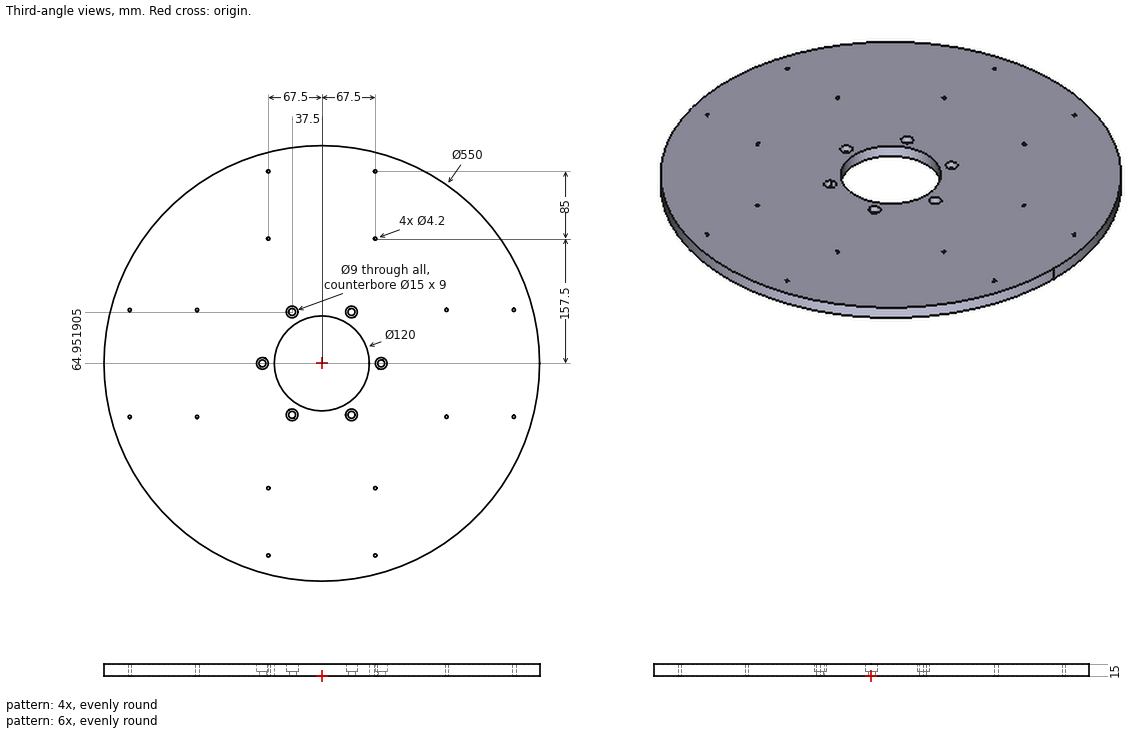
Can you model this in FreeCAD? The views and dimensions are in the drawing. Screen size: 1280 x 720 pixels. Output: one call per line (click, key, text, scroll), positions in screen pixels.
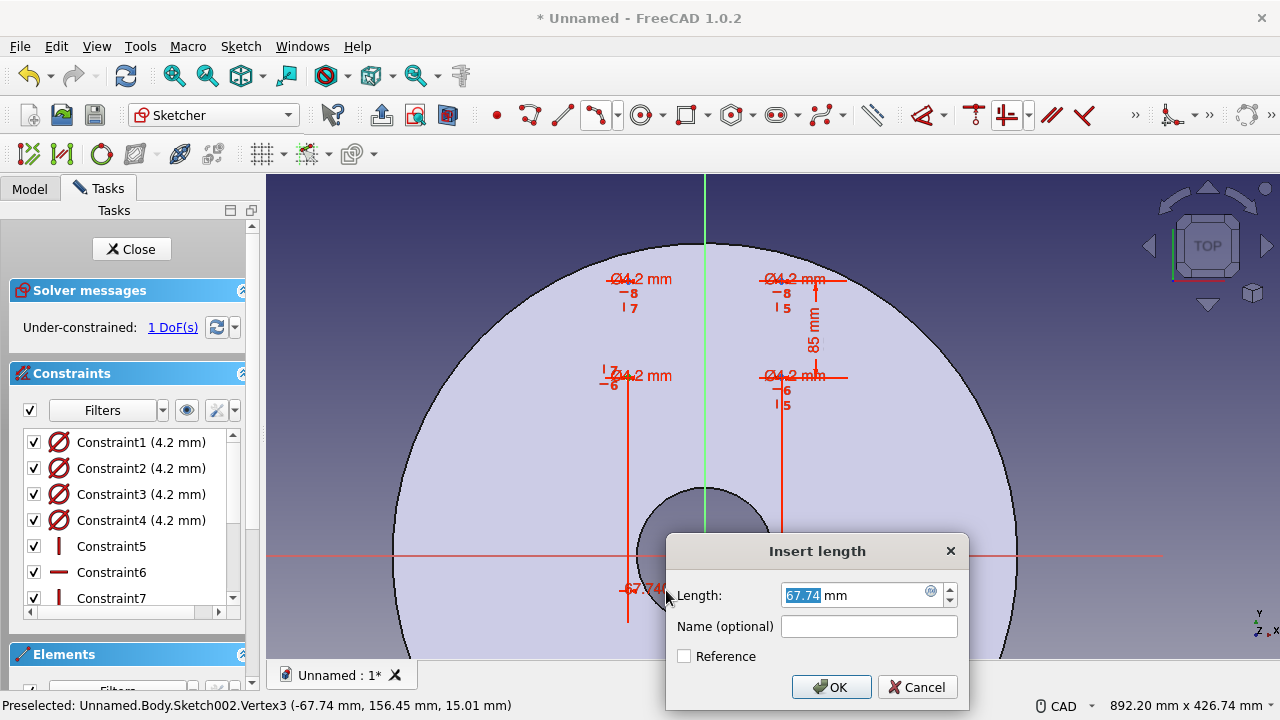
text(67.5)
key(Return)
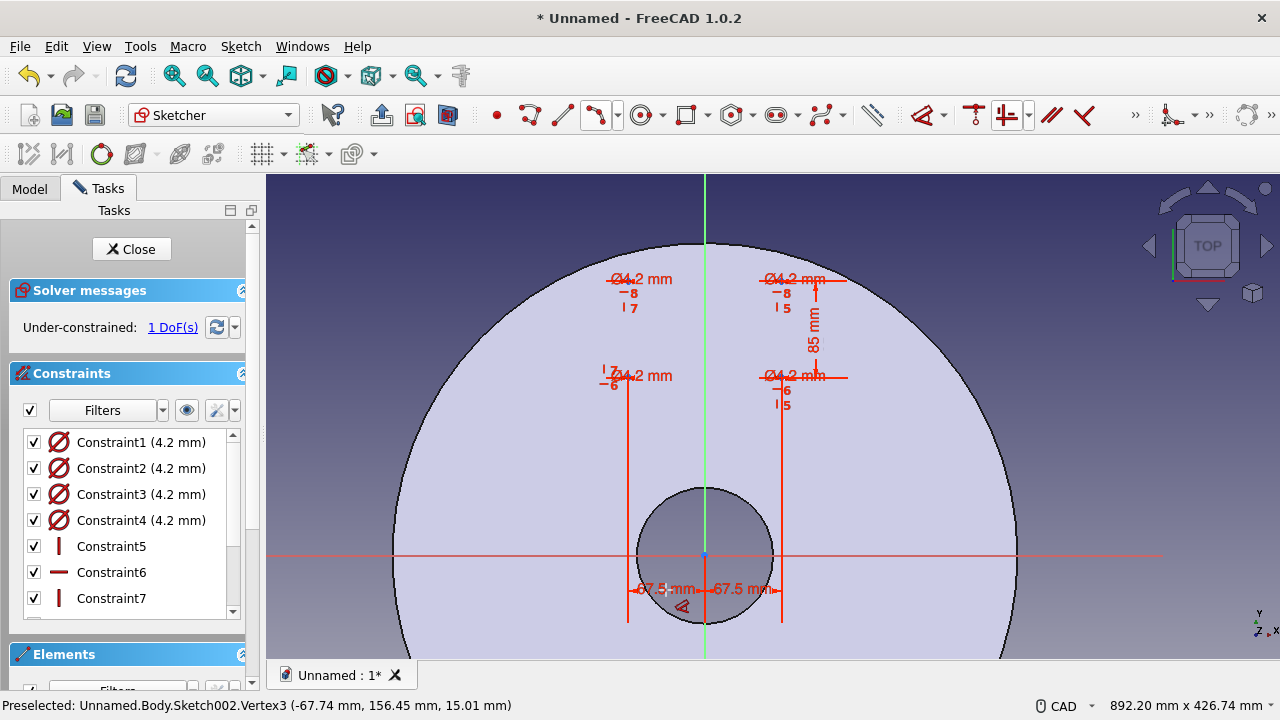
click(782, 378)
click(816, 467)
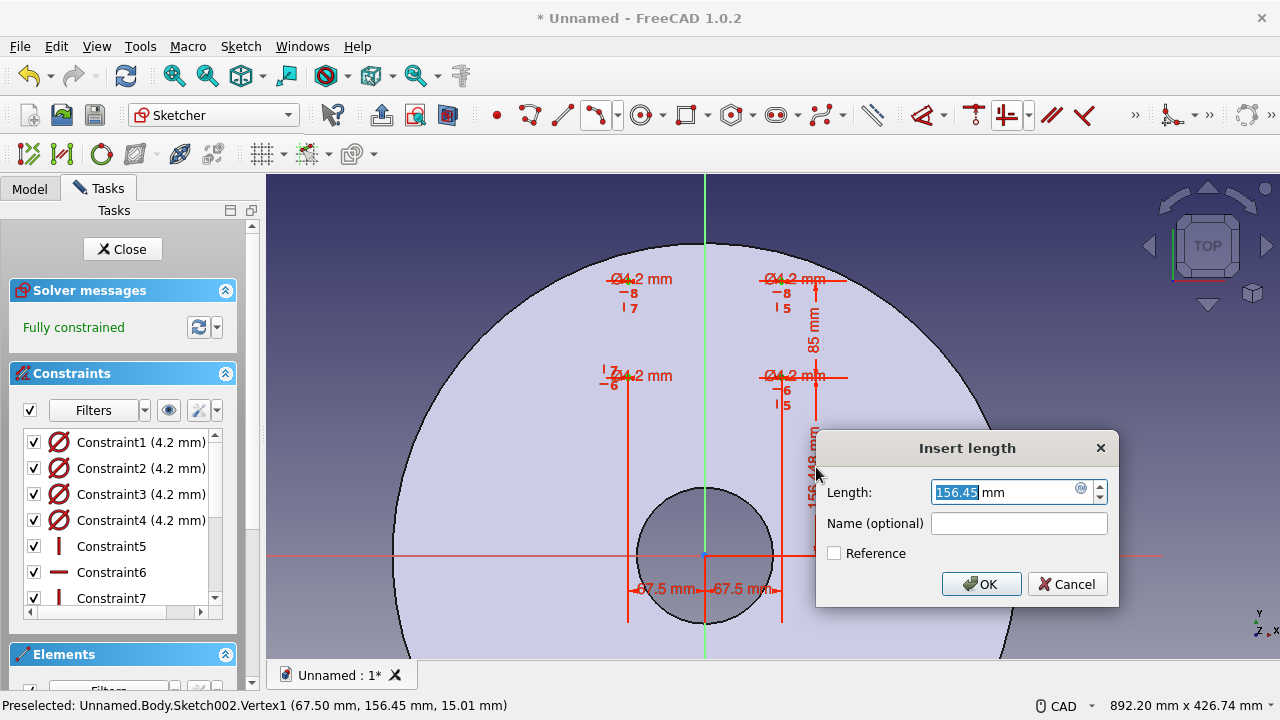
text(157.5)
key(Return)
key(Escape)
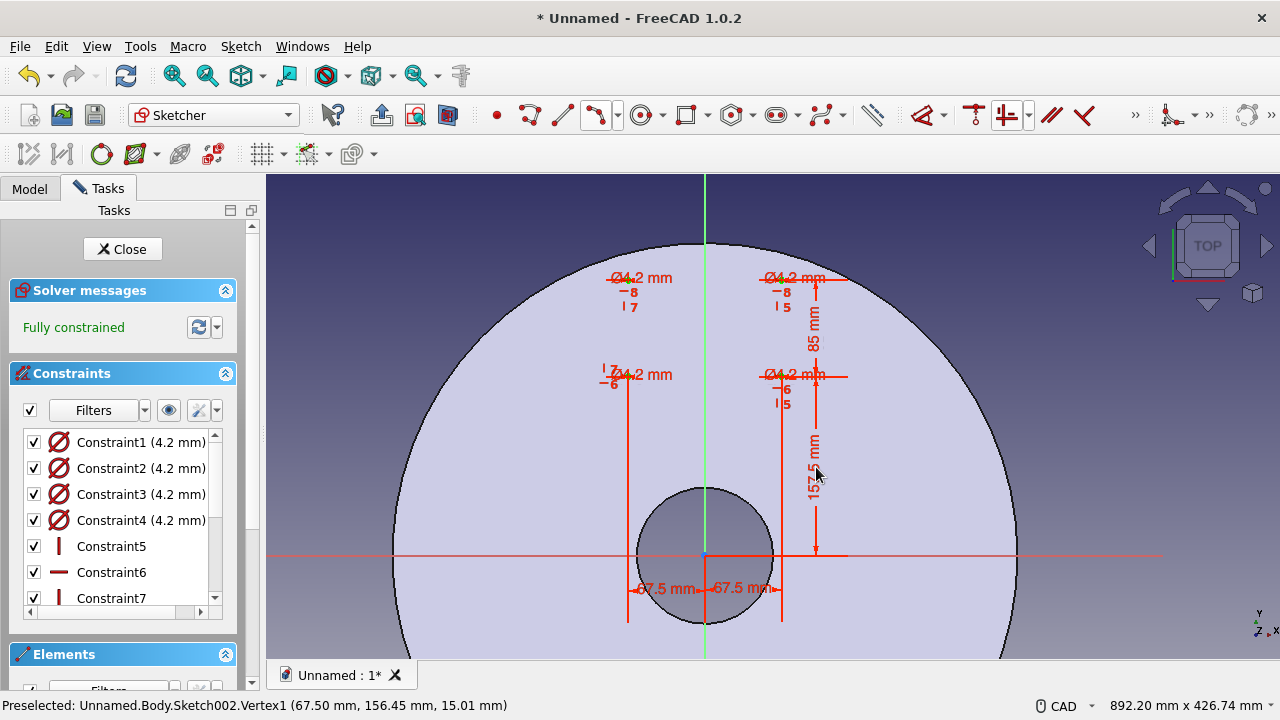
click(123, 249)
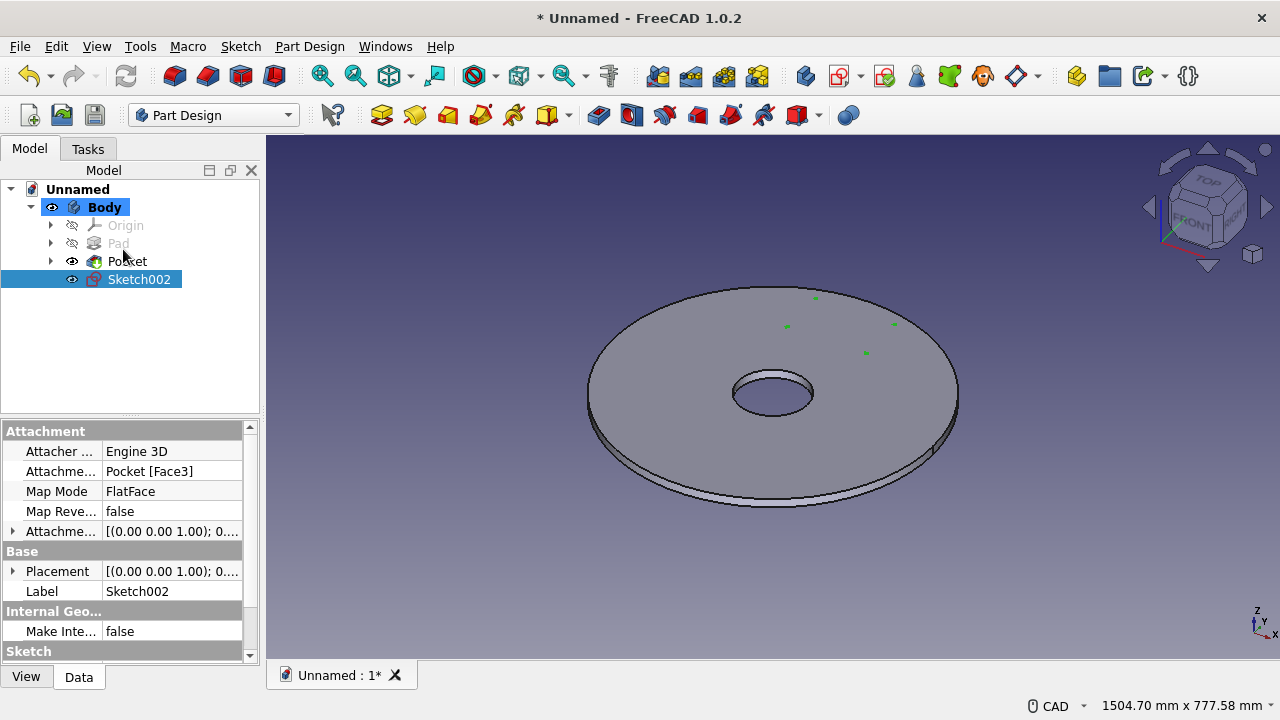
click(599, 116)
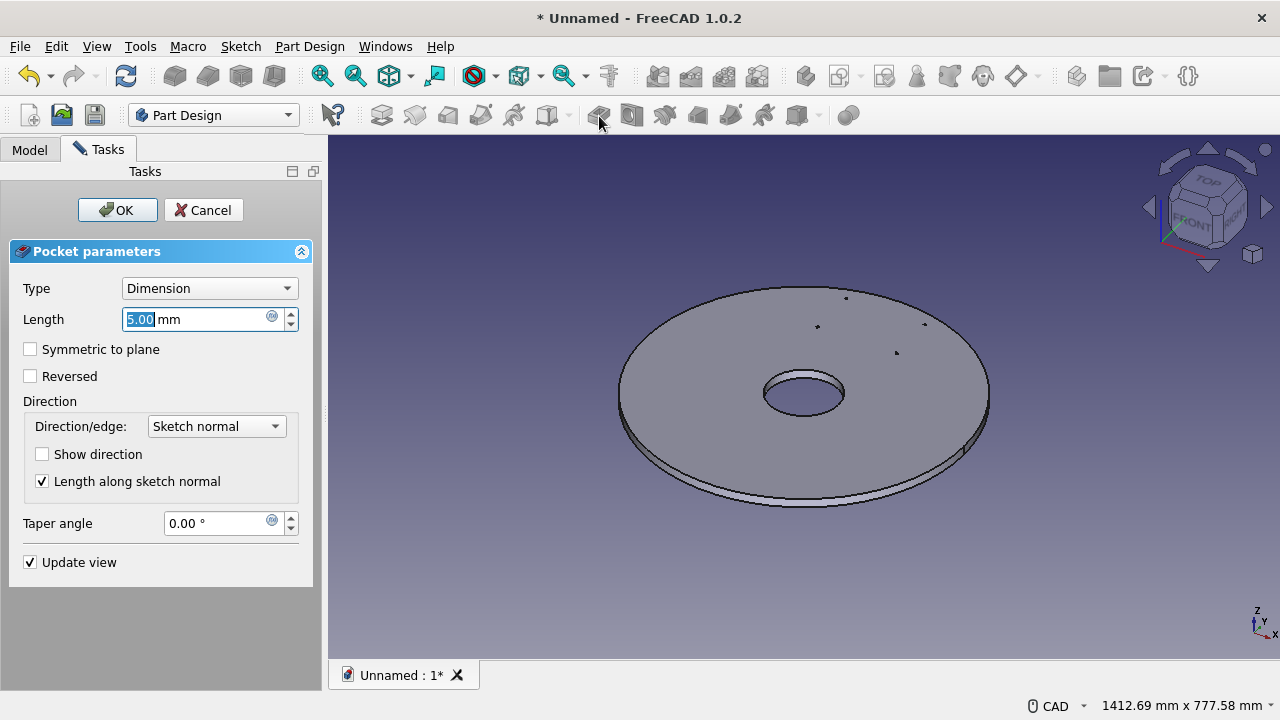
click(210, 288)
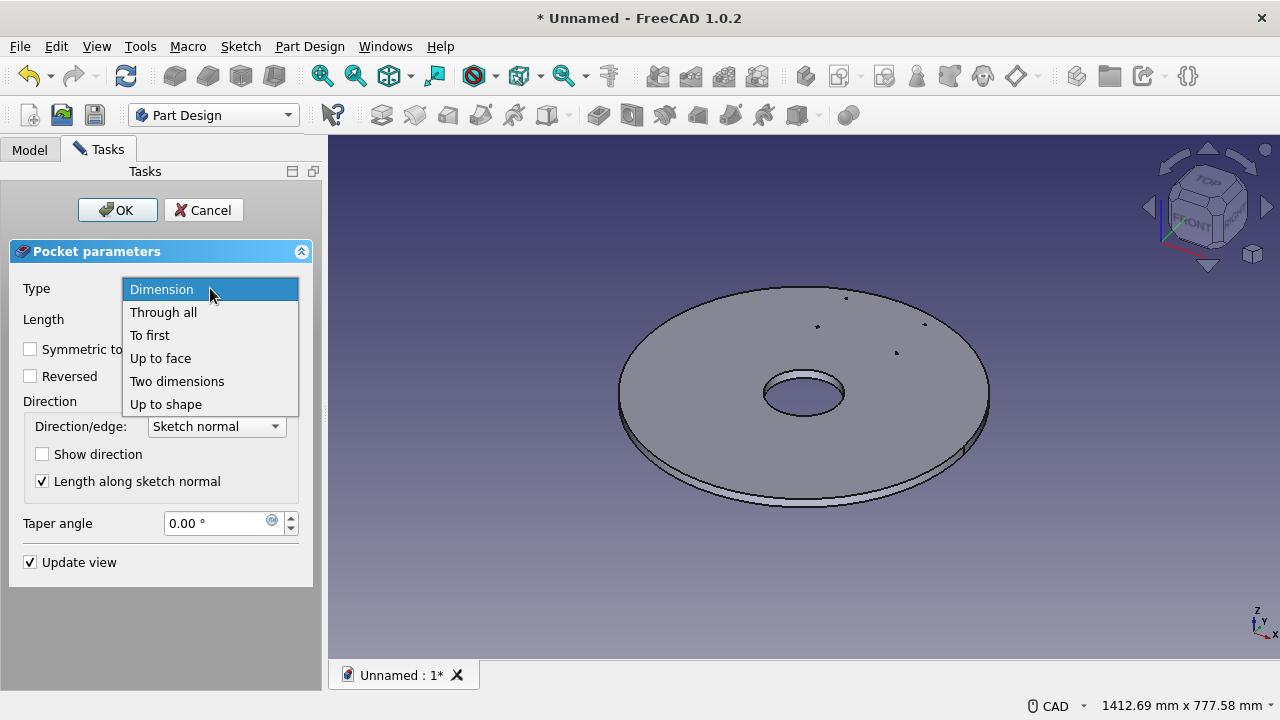
click(208, 312)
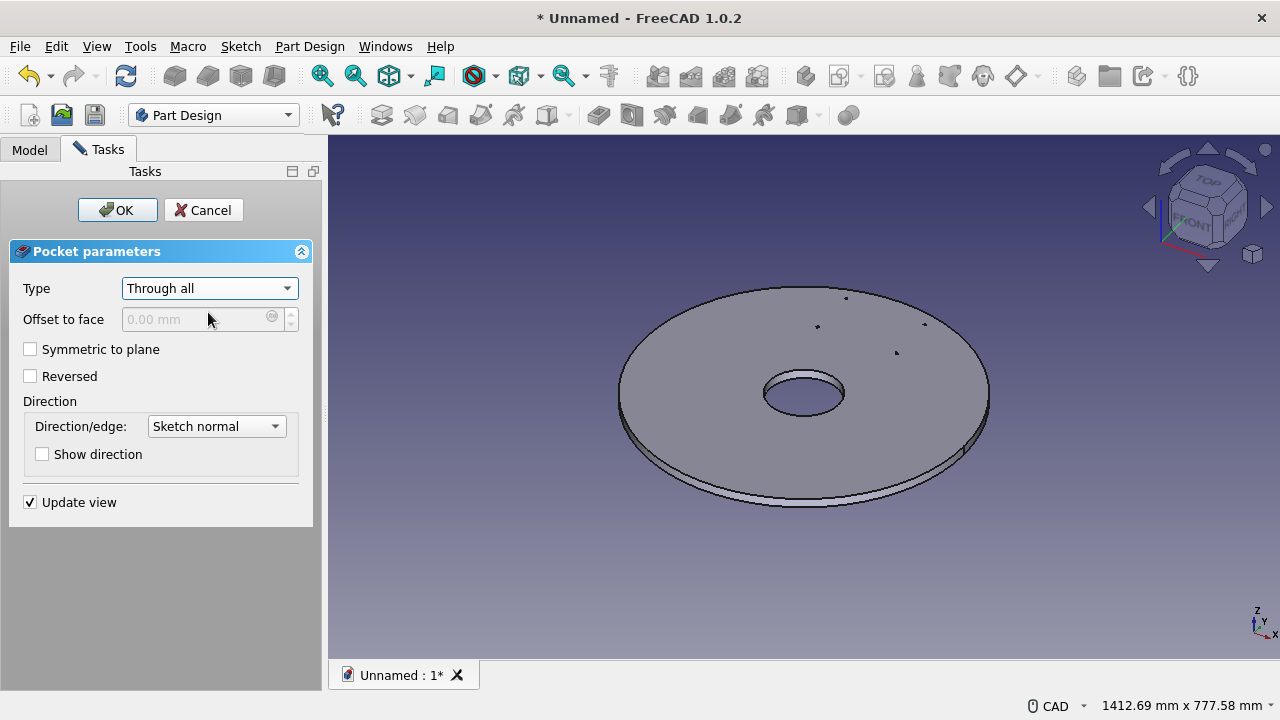
click(118, 210)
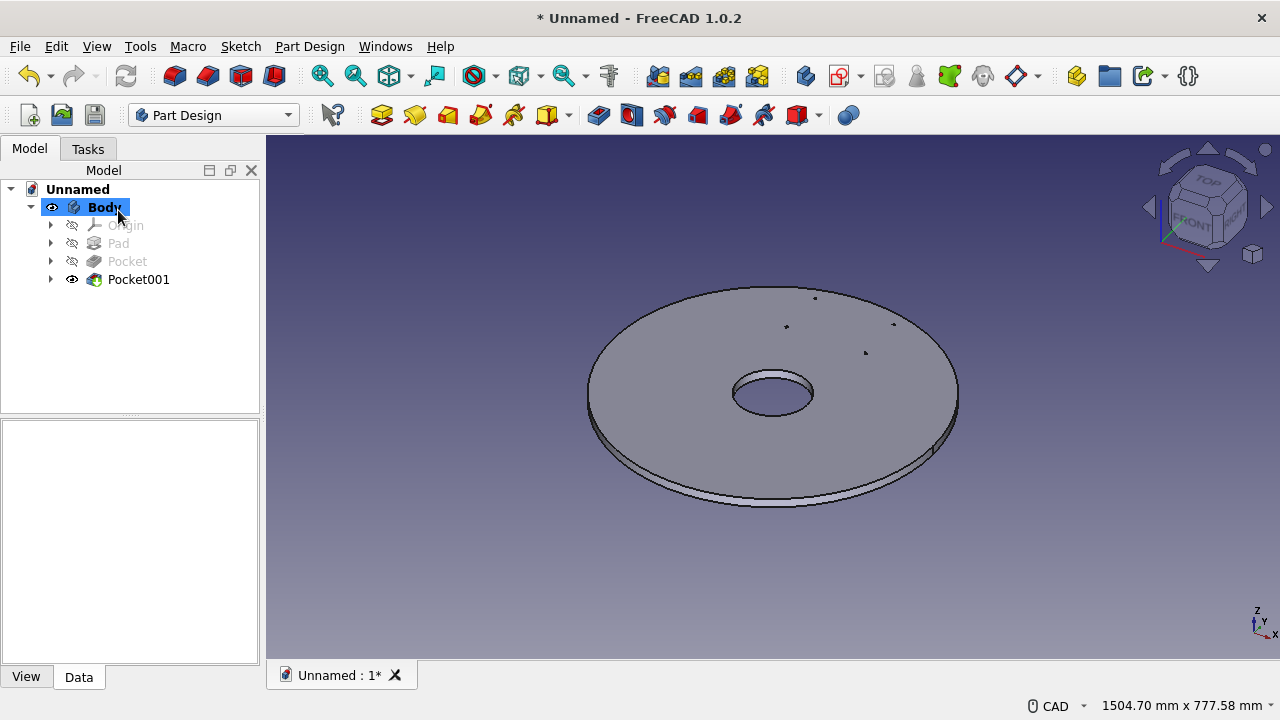
click(117, 279)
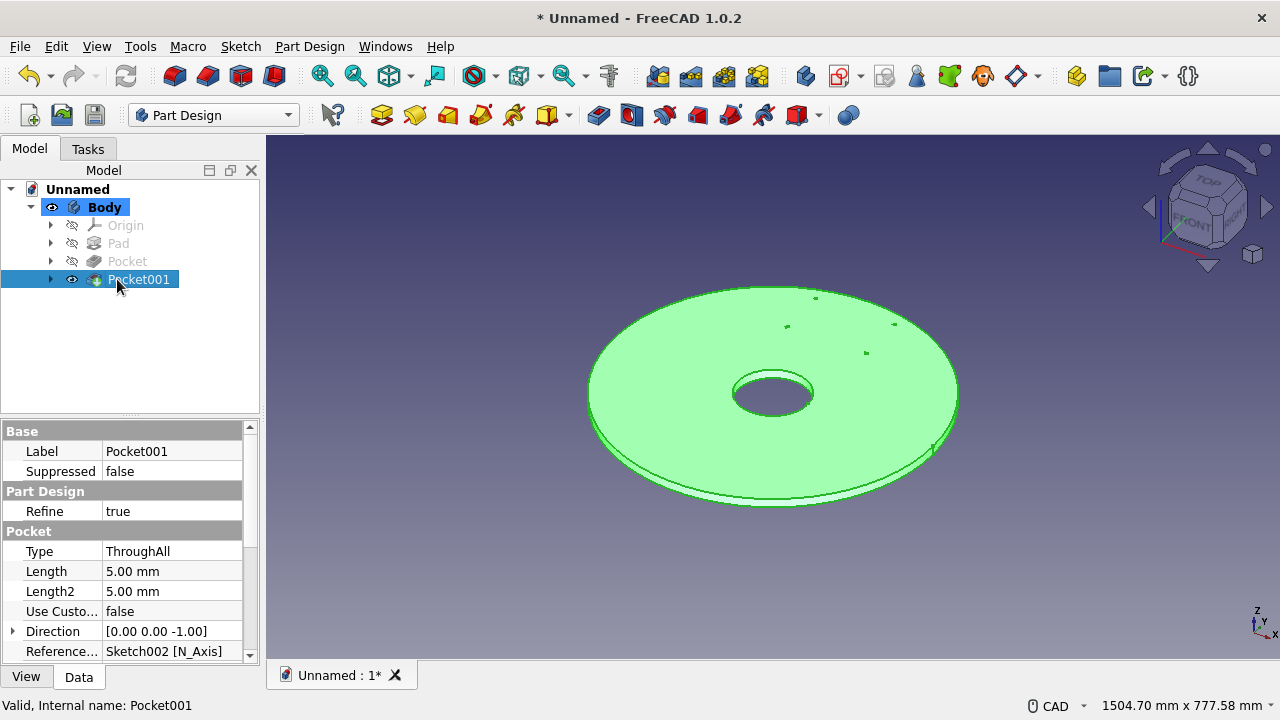
click(724, 76)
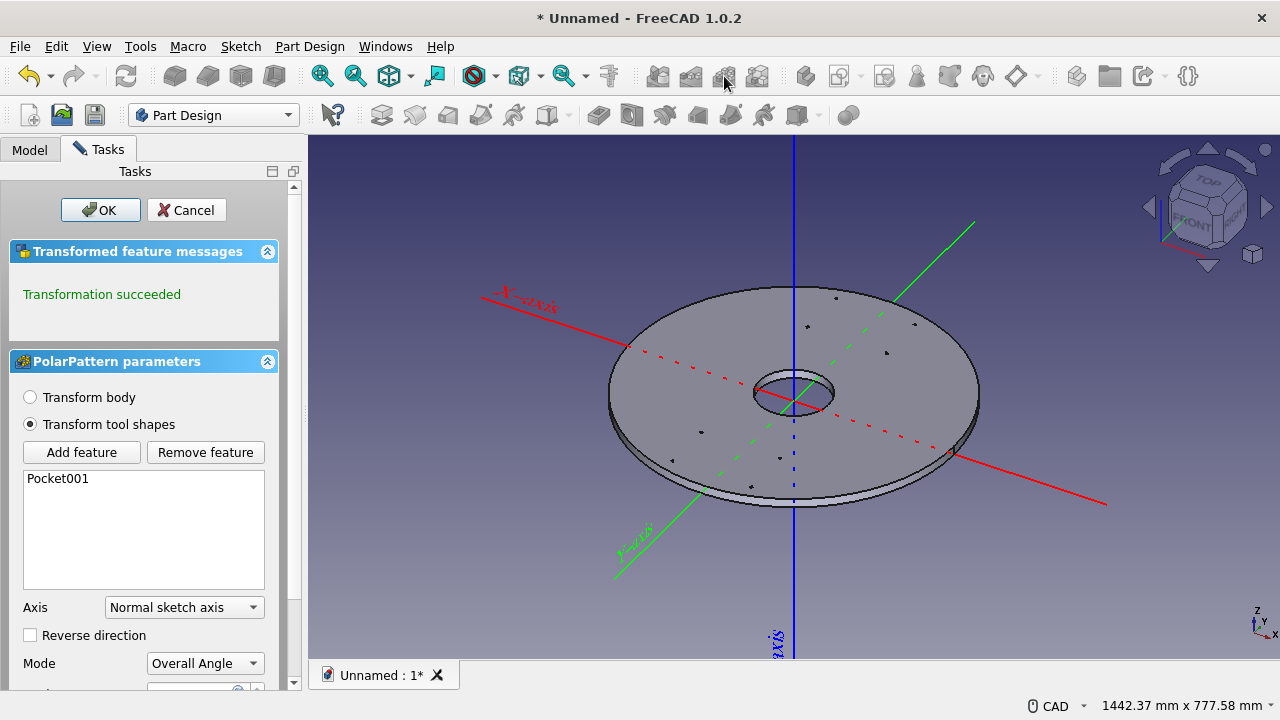
click(185, 608)